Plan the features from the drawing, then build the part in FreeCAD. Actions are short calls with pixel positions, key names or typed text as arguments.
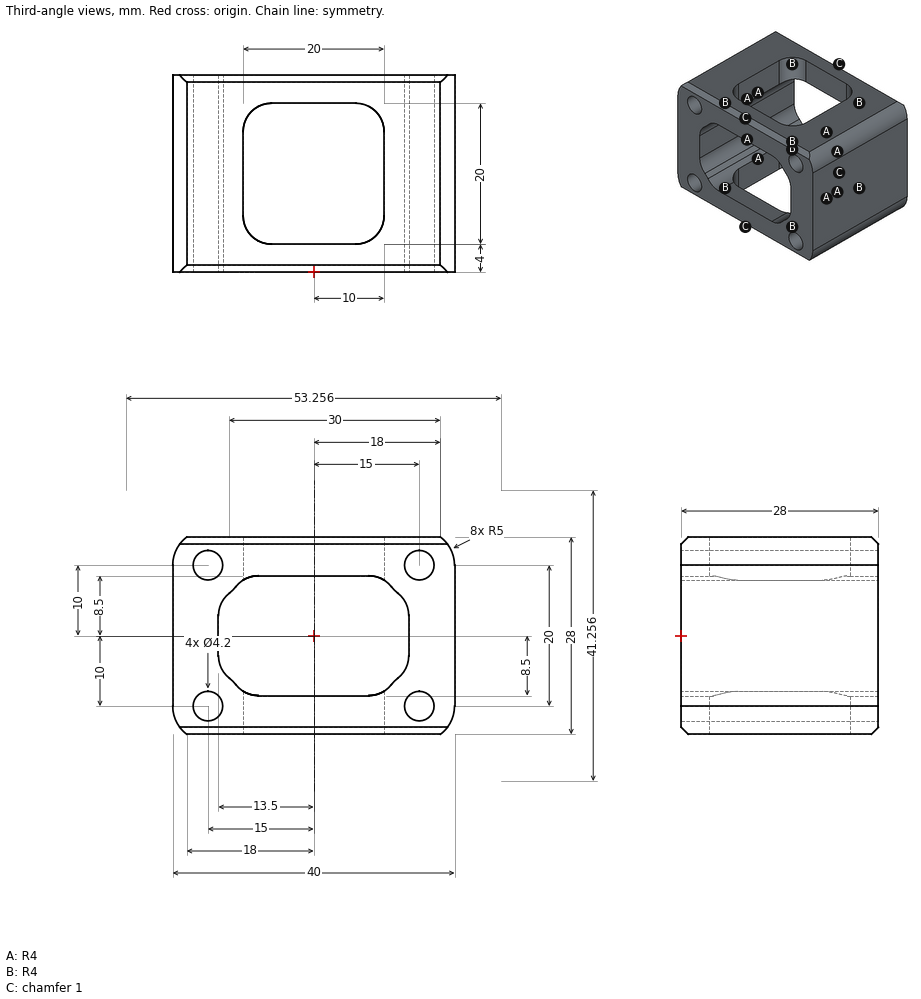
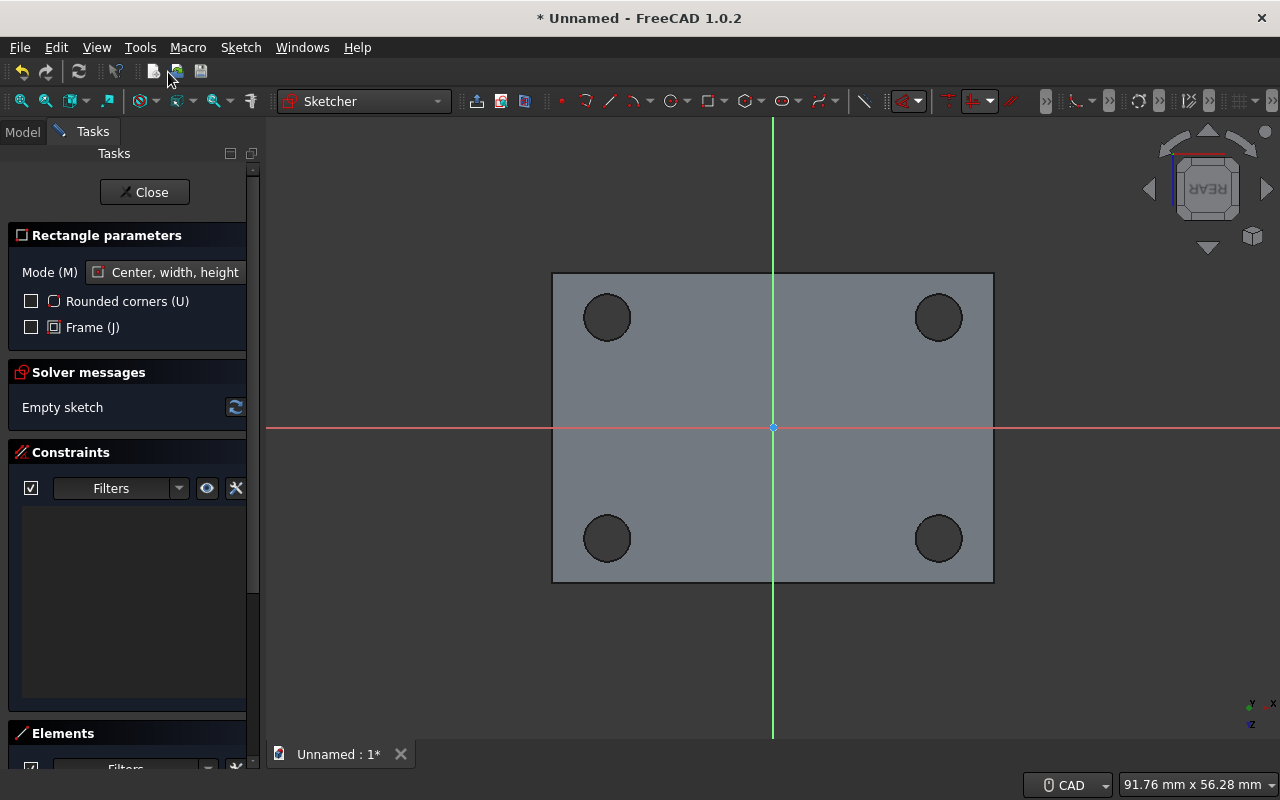
click(773, 428)
click(1067, 200)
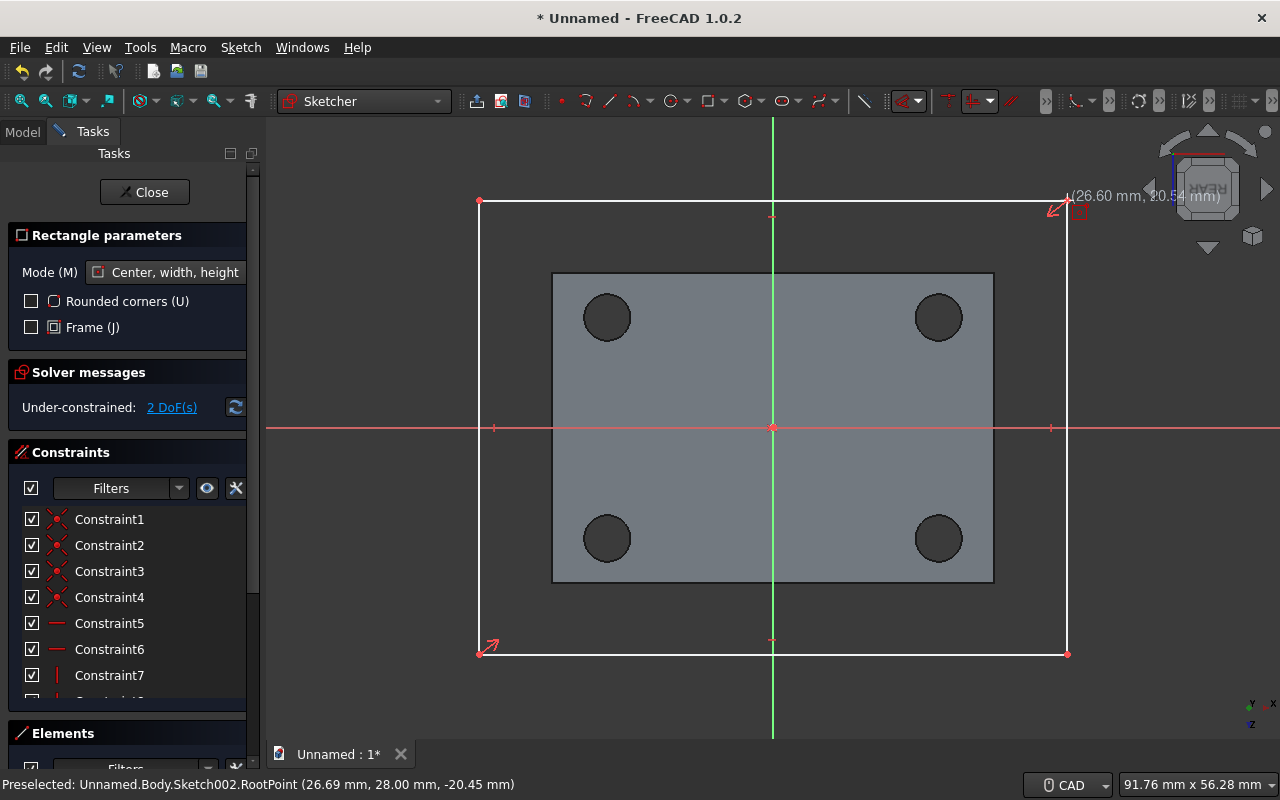
click(610, 102)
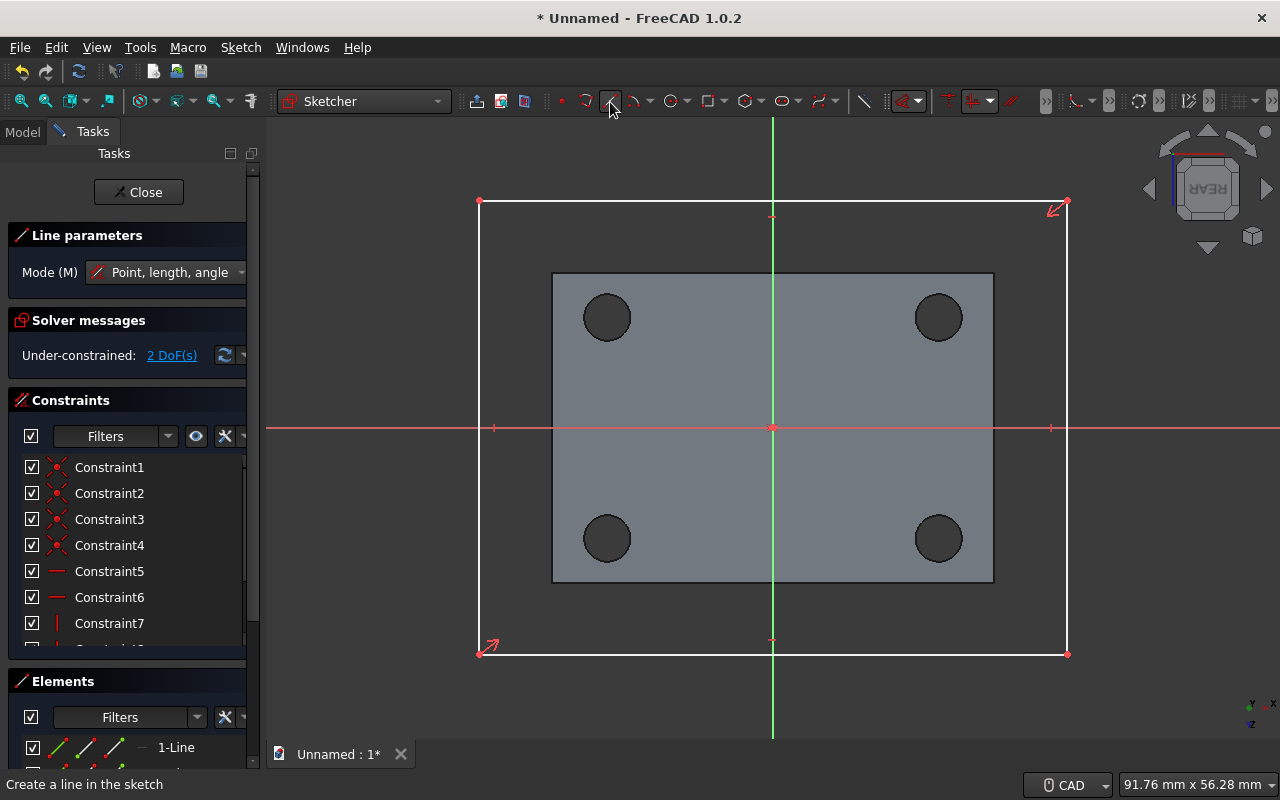
click(624, 370)
click(624, 486)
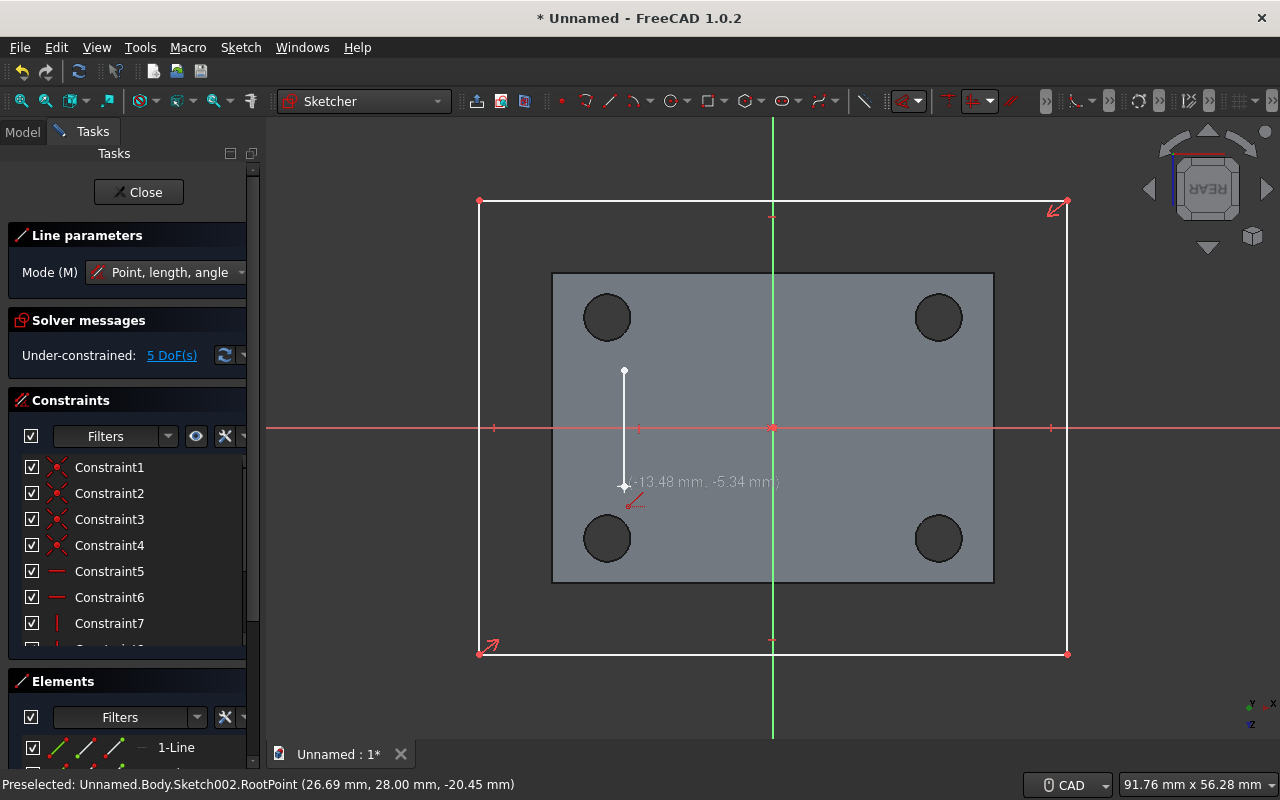
click(660, 522)
click(886, 522)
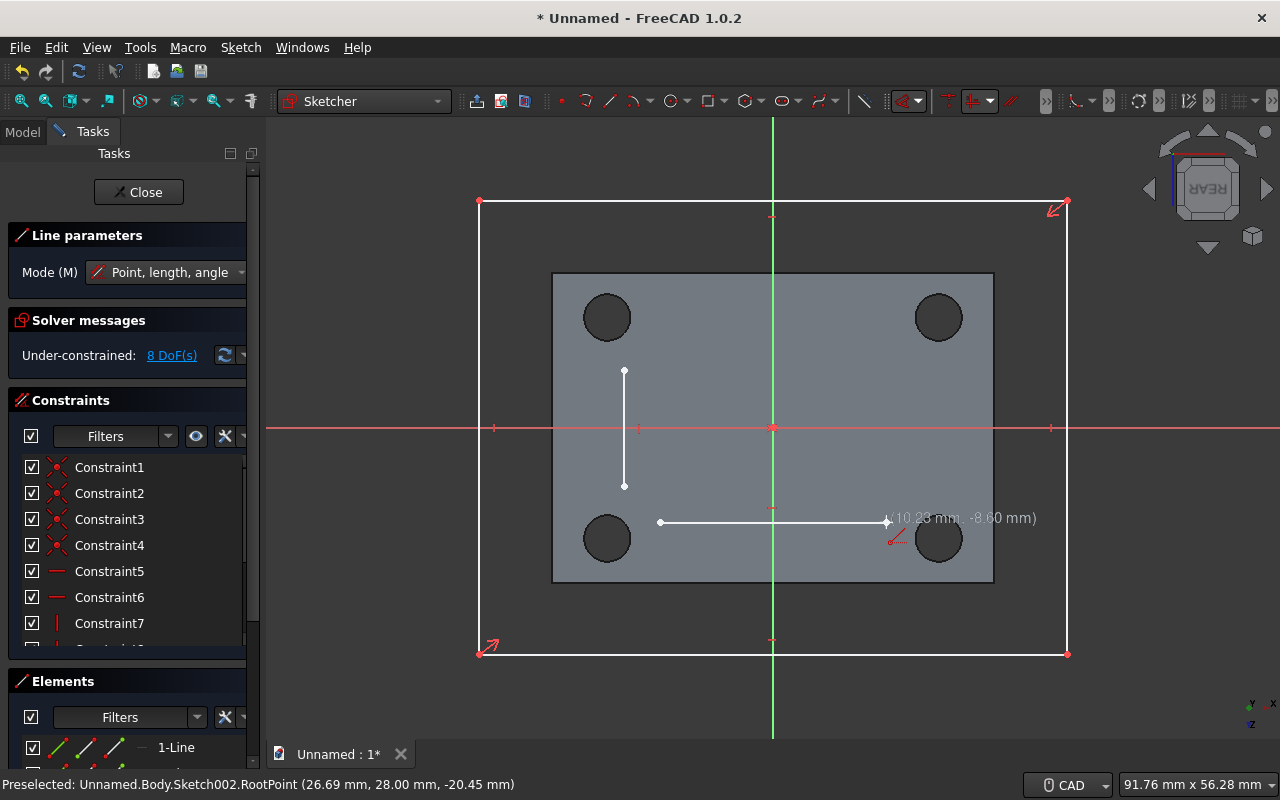
click(922, 486)
click(922, 370)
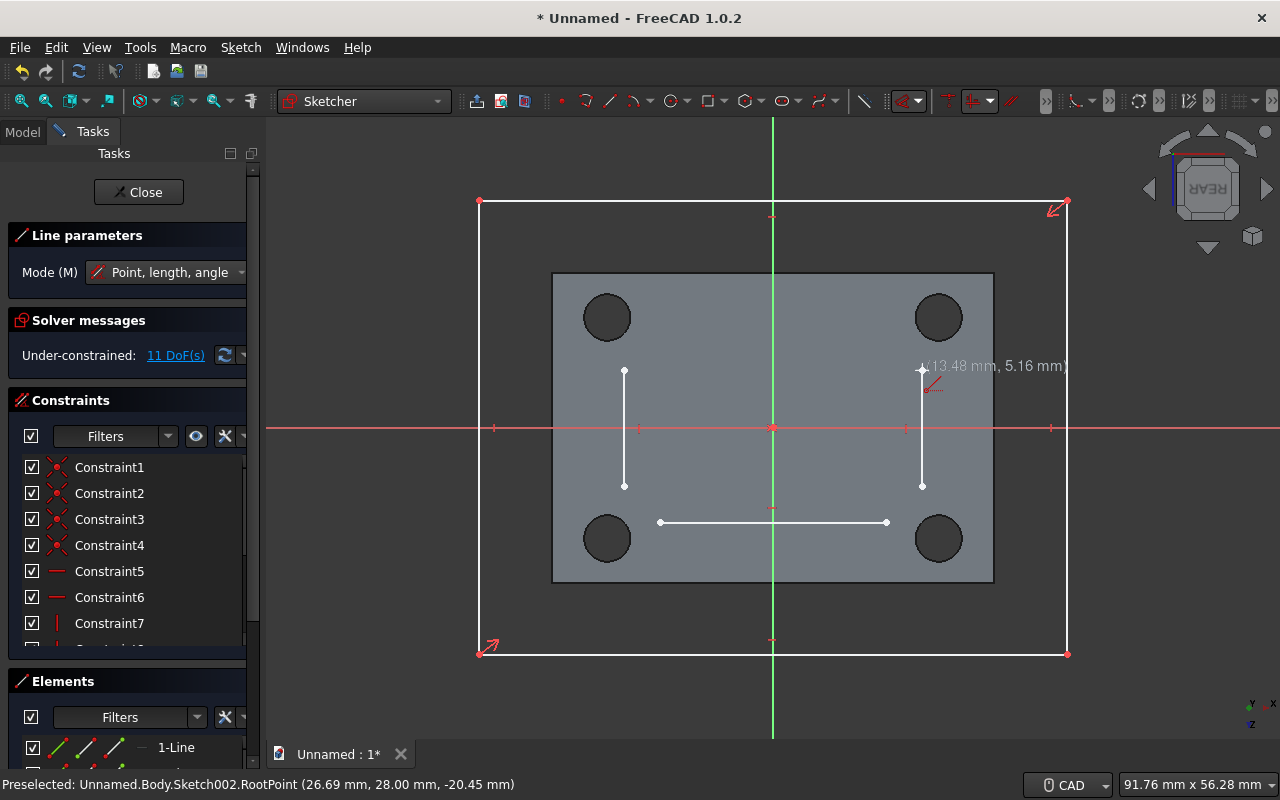
click(886, 334)
click(660, 334)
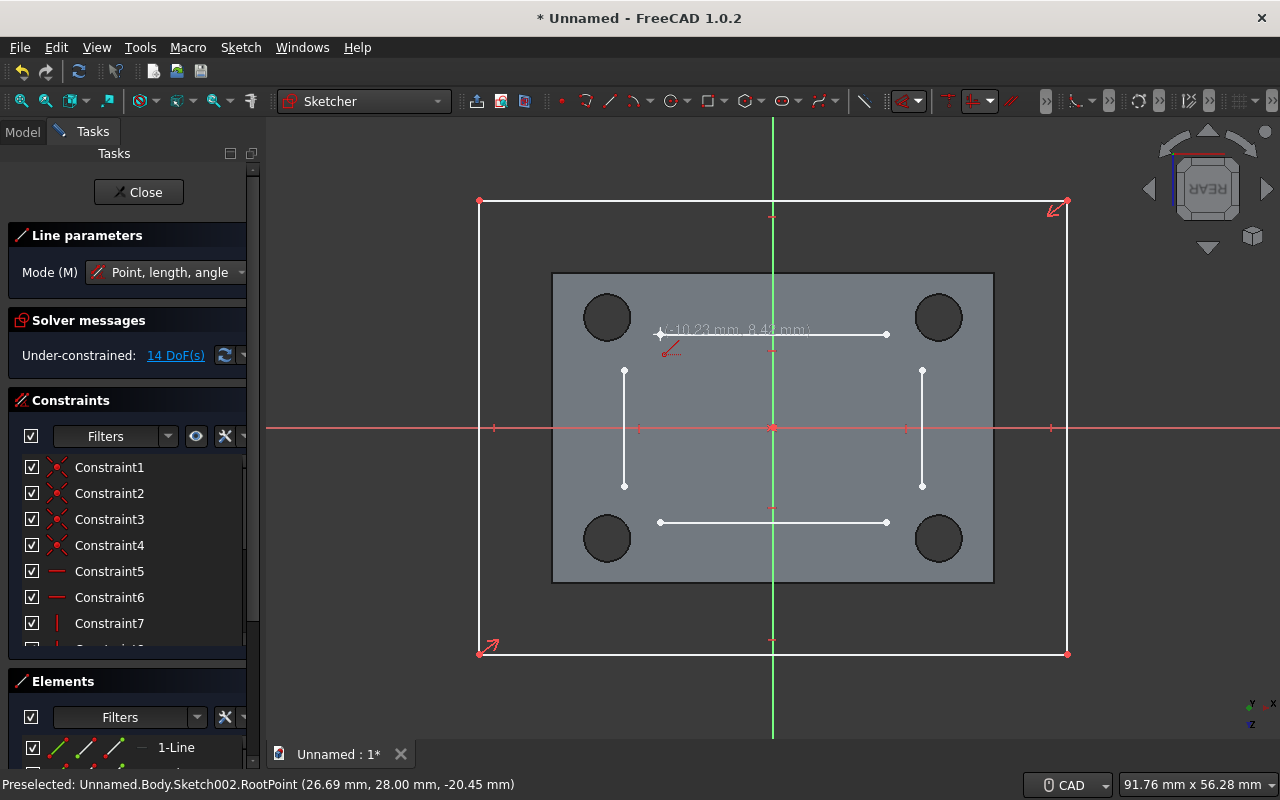
key(g)
key(3)
key(a)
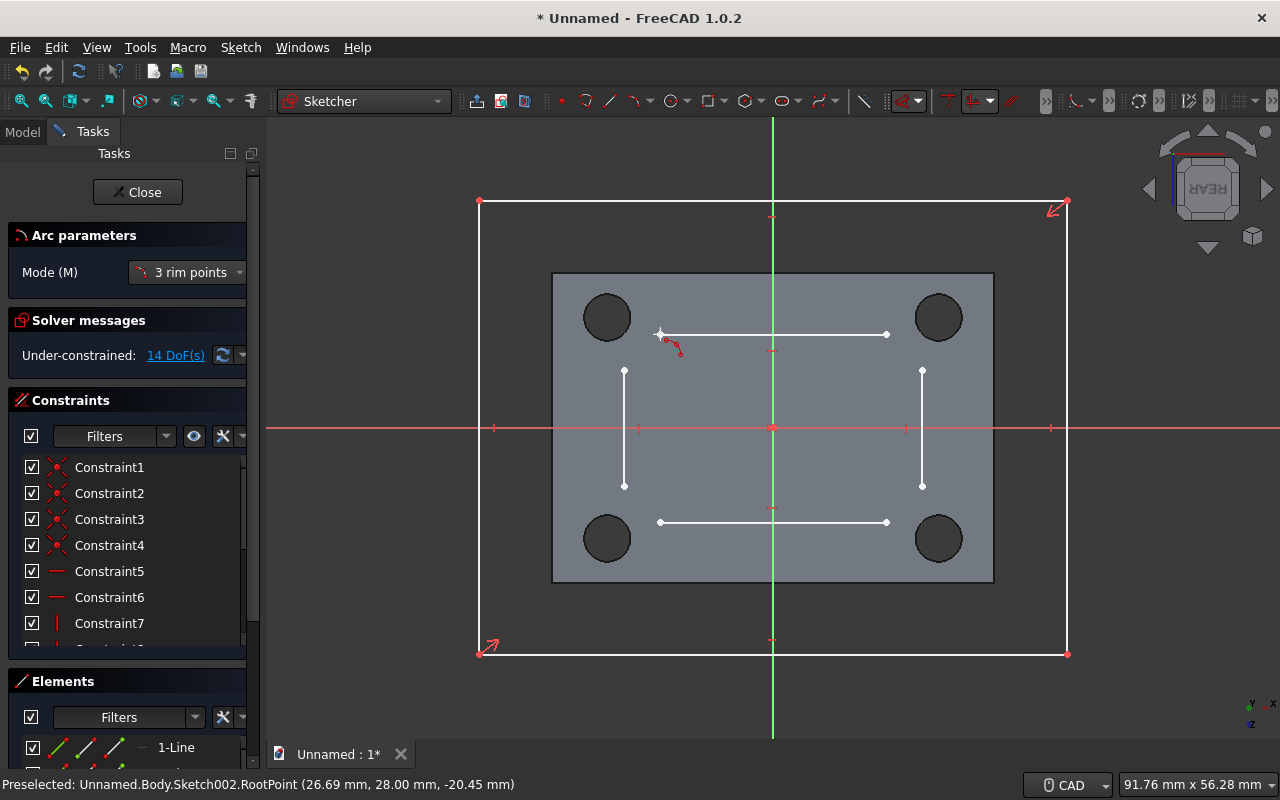
click(624, 487)
click(660, 523)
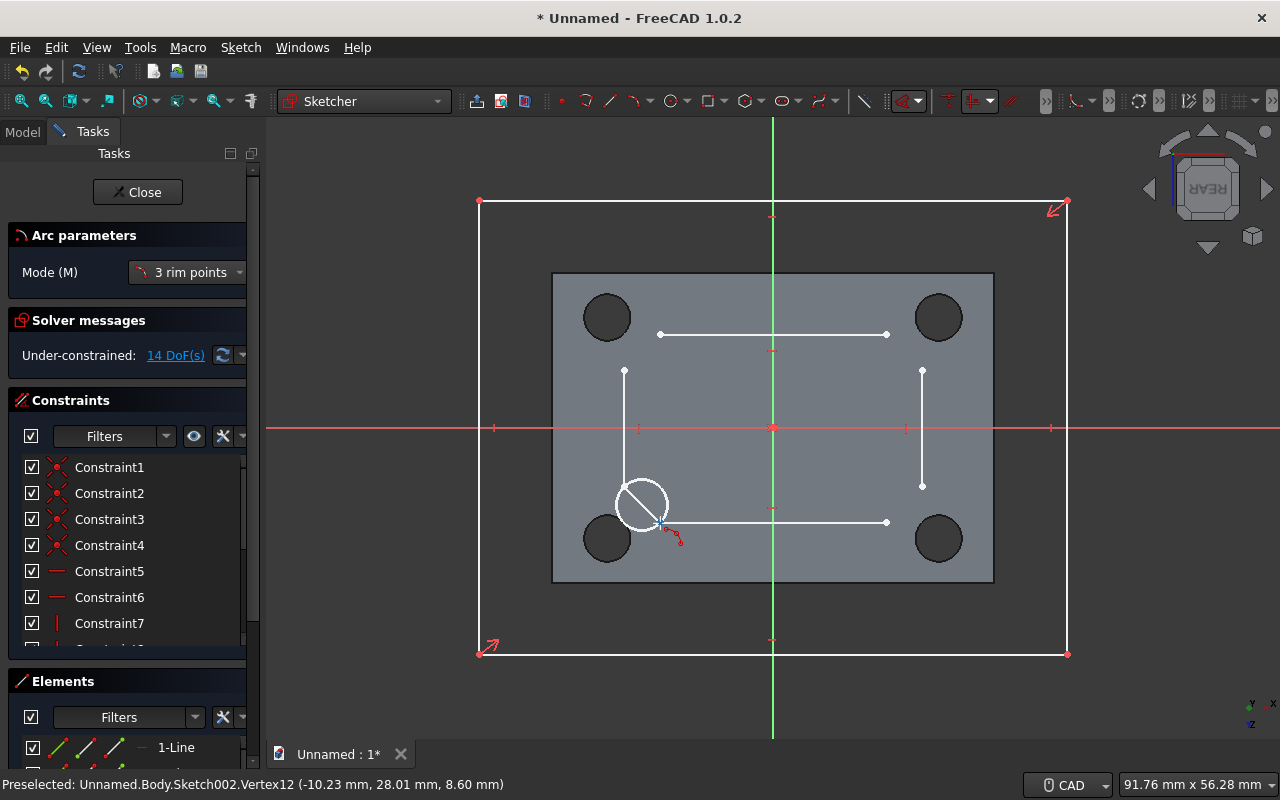
scroll(646, 499, up, 5)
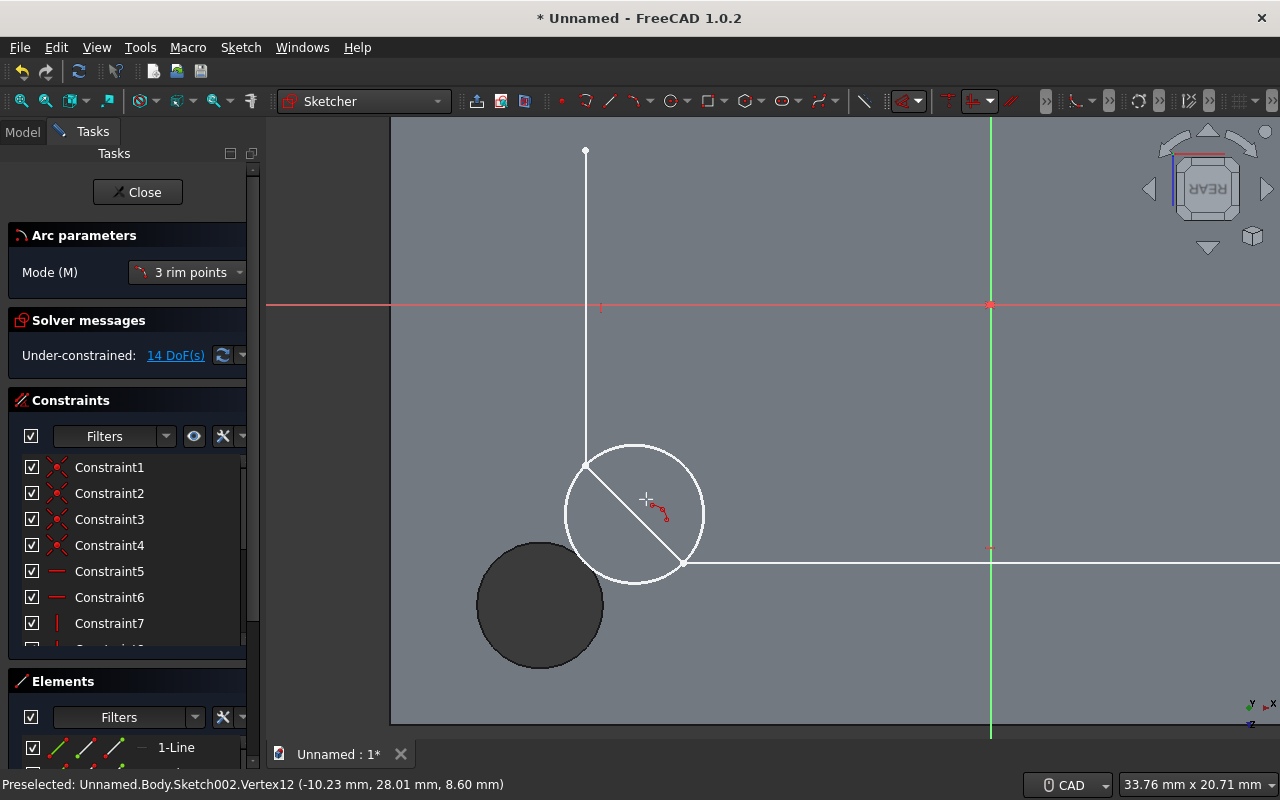
click(646, 499)